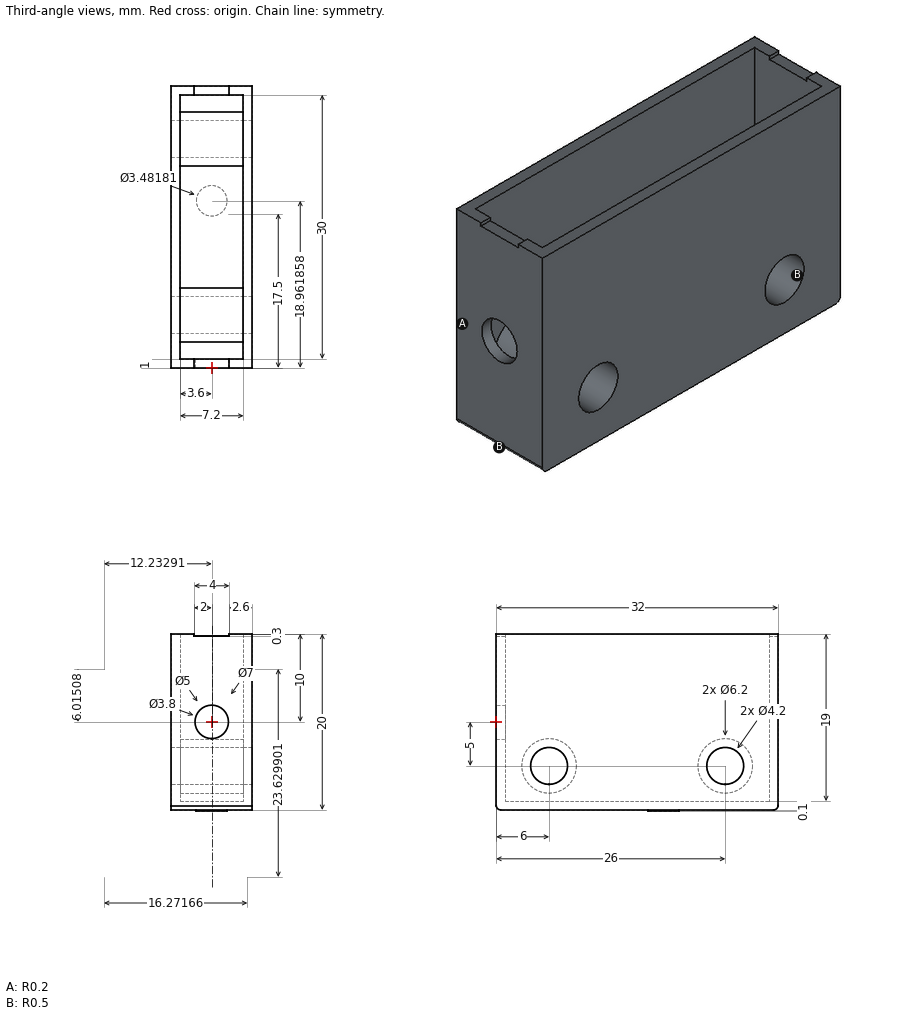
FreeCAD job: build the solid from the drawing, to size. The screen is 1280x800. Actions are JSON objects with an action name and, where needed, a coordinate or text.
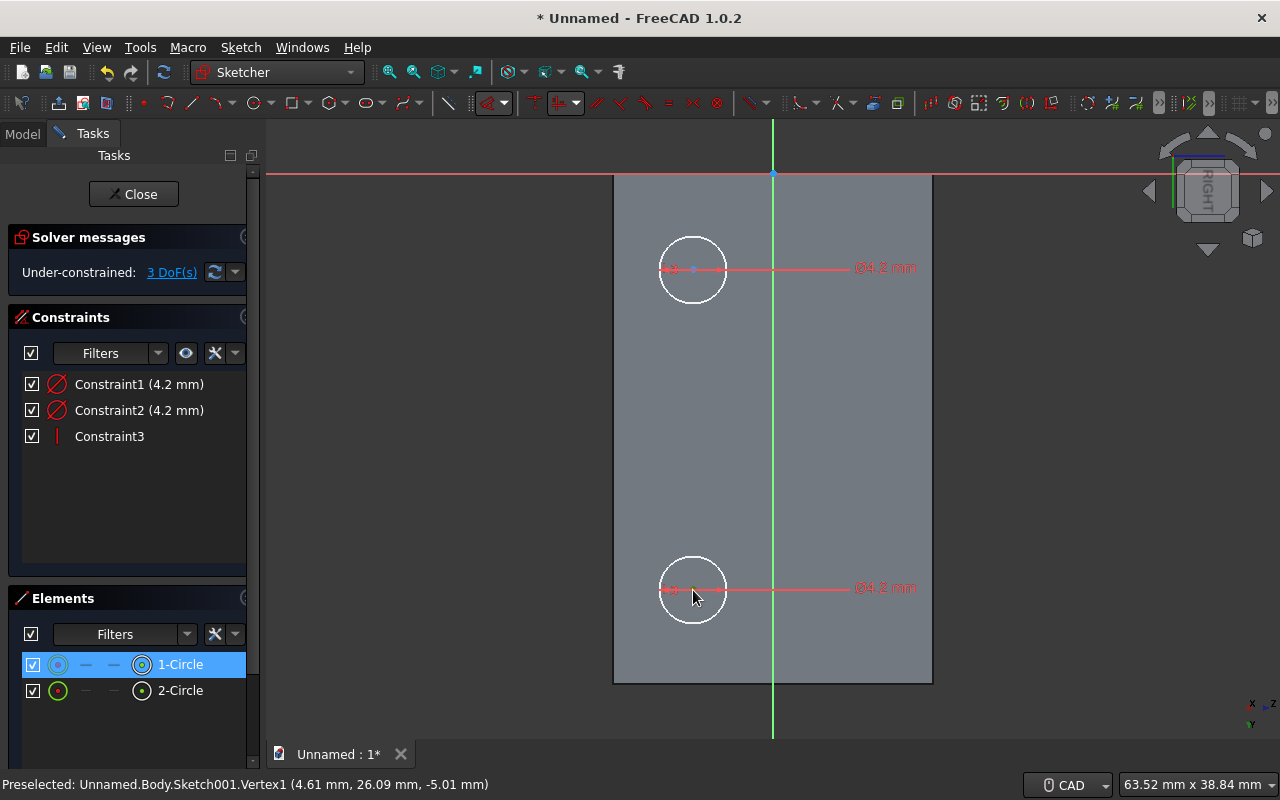
{"action": "key", "text": "l"}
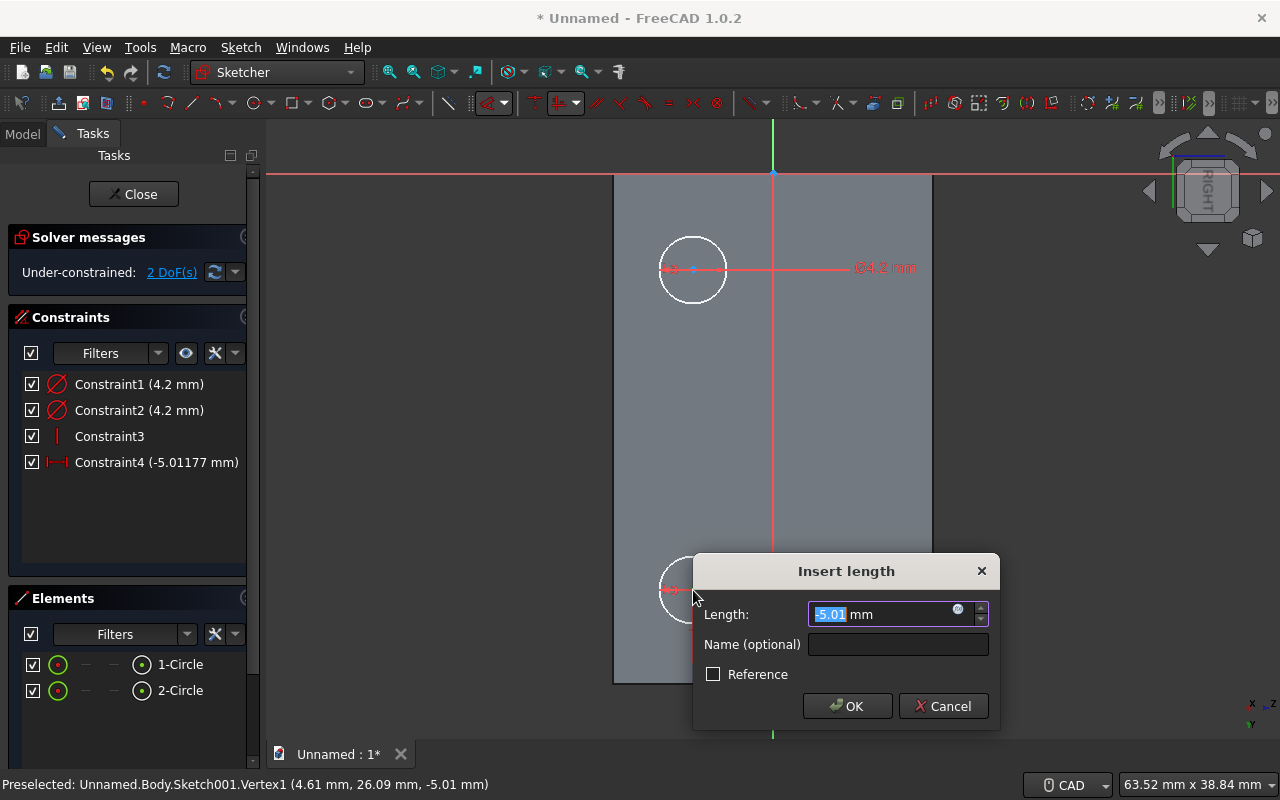
{"action": "type", "text": "-5"}
{"action": "key", "text": "Return"}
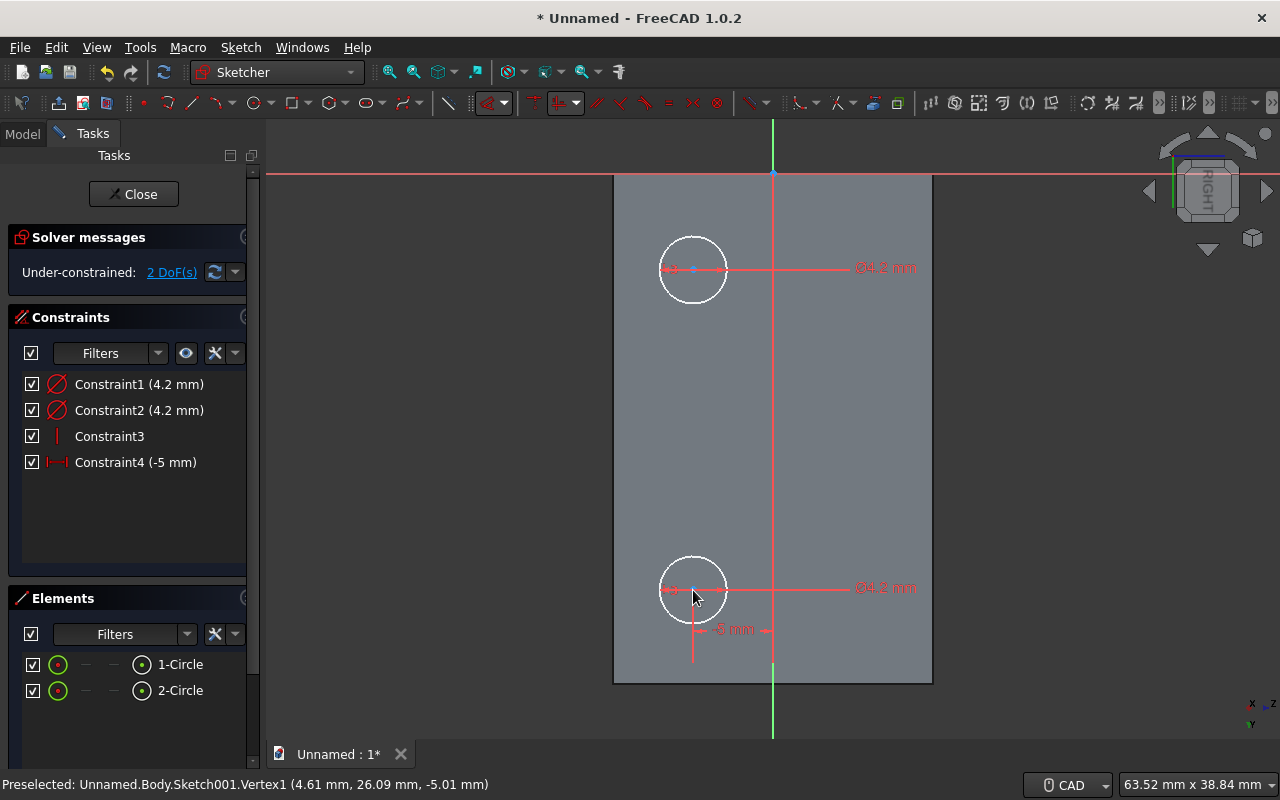
{"action": "left_click", "coordinate": [693, 270]}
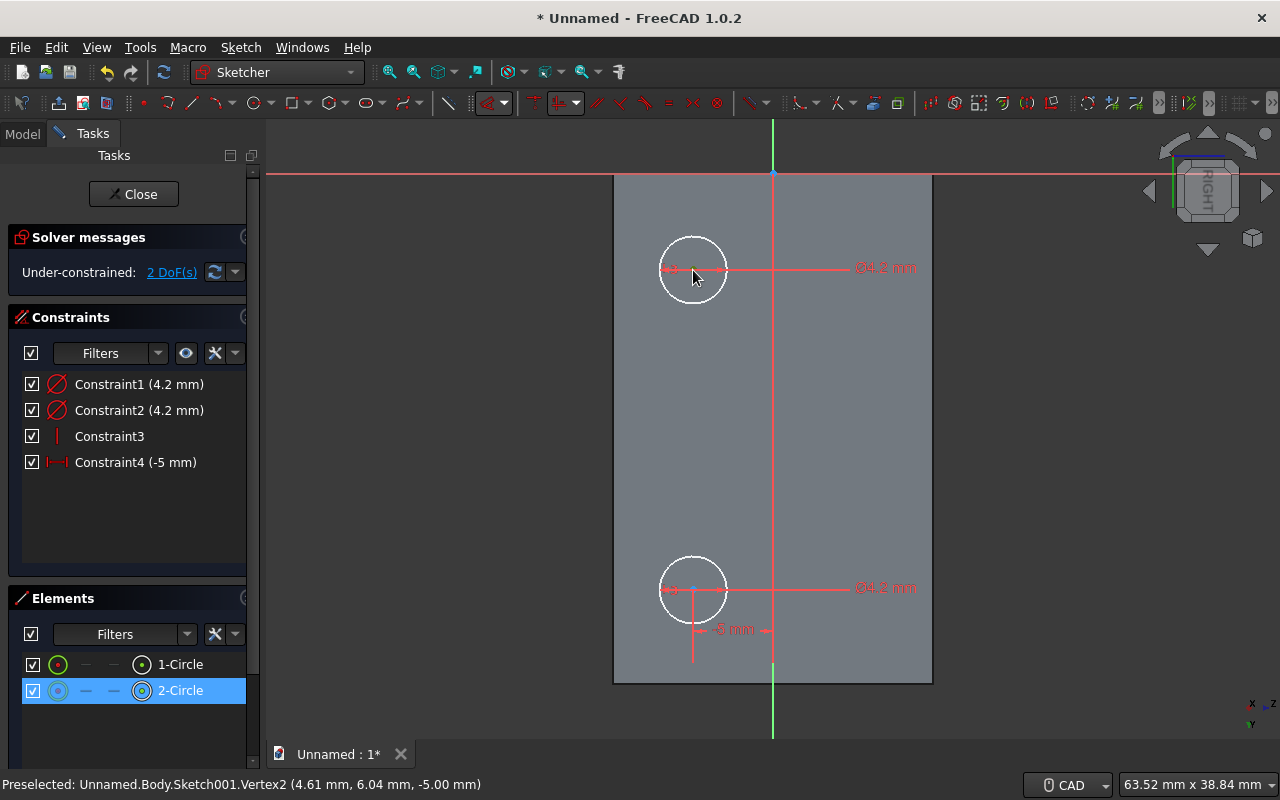
{"action": "left_click", "coordinate": [506, 104]}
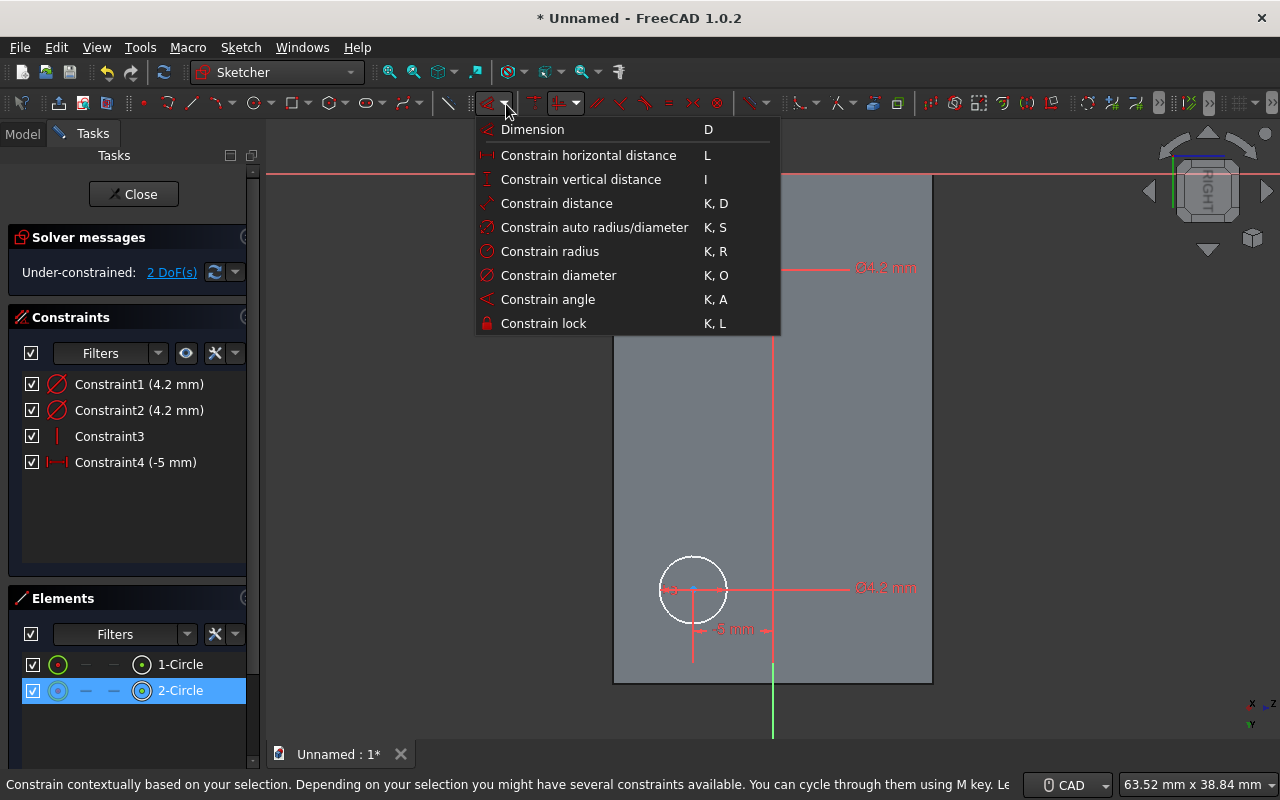
{"action": "left_click", "coordinate": [628, 179]}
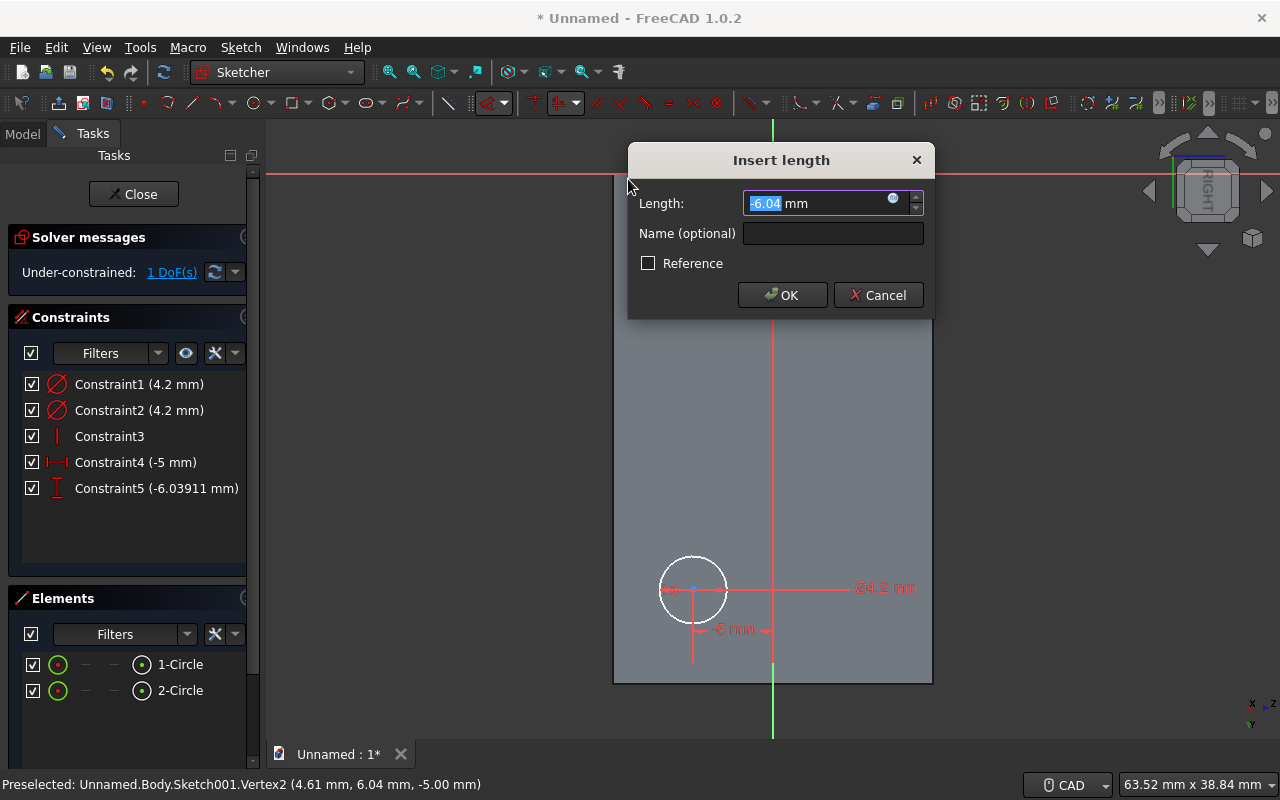
{"action": "type", "text": "-6"}
{"action": "key", "text": "Return"}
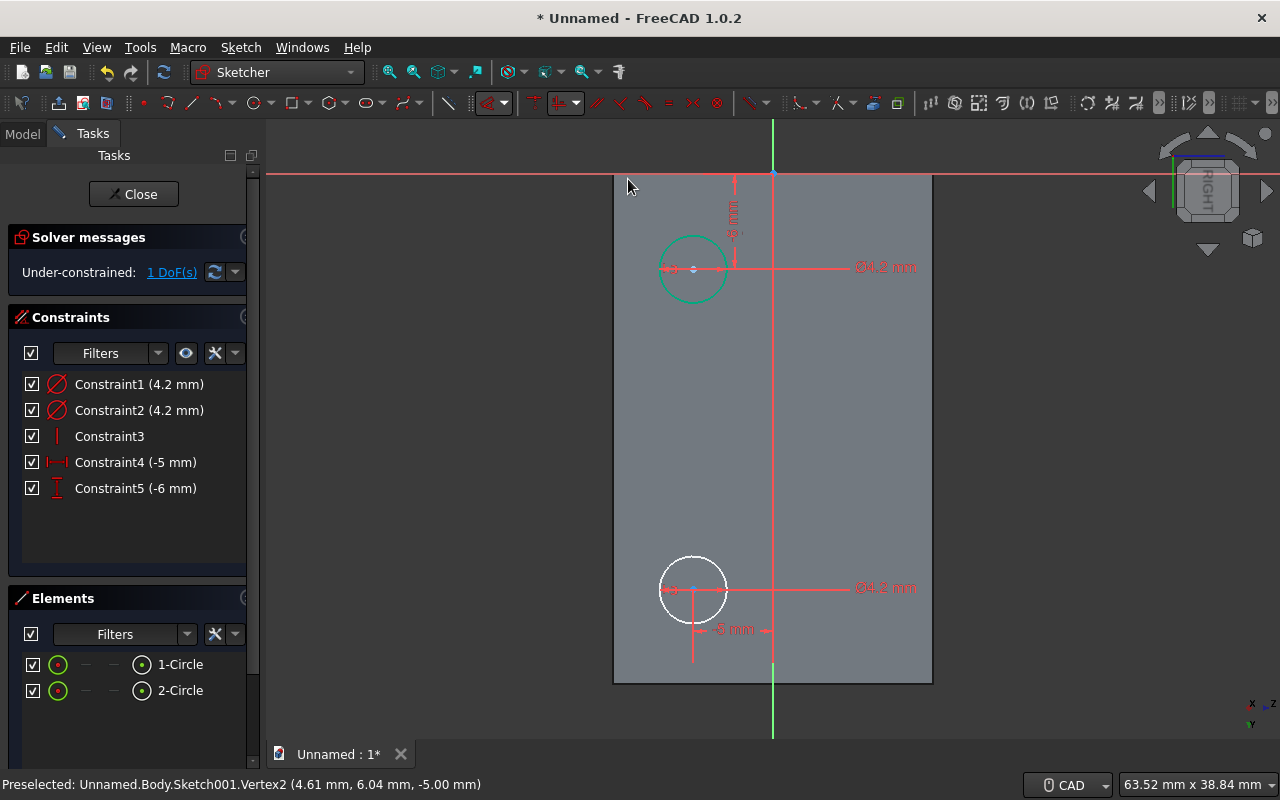
{"action": "left_click", "coordinate": [693, 590]}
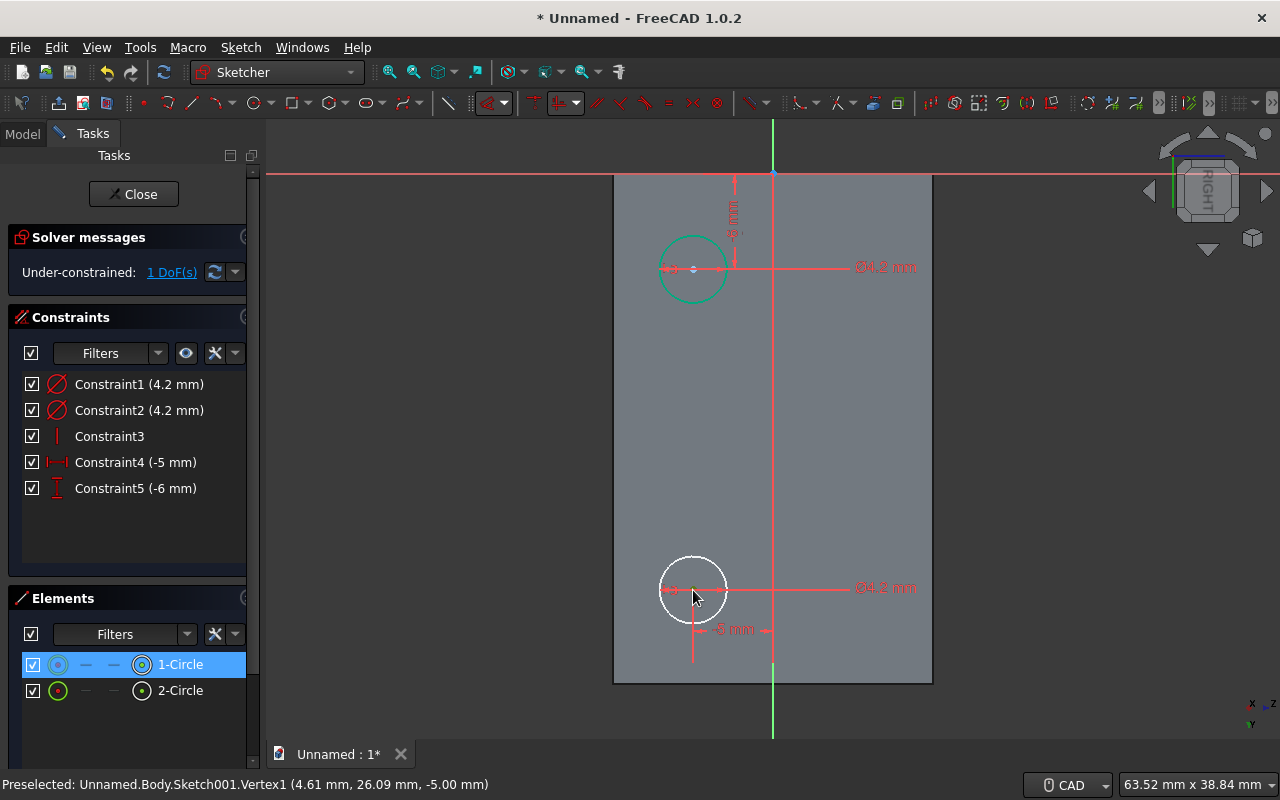
{"action": "left_click", "coordinate": [506, 104]}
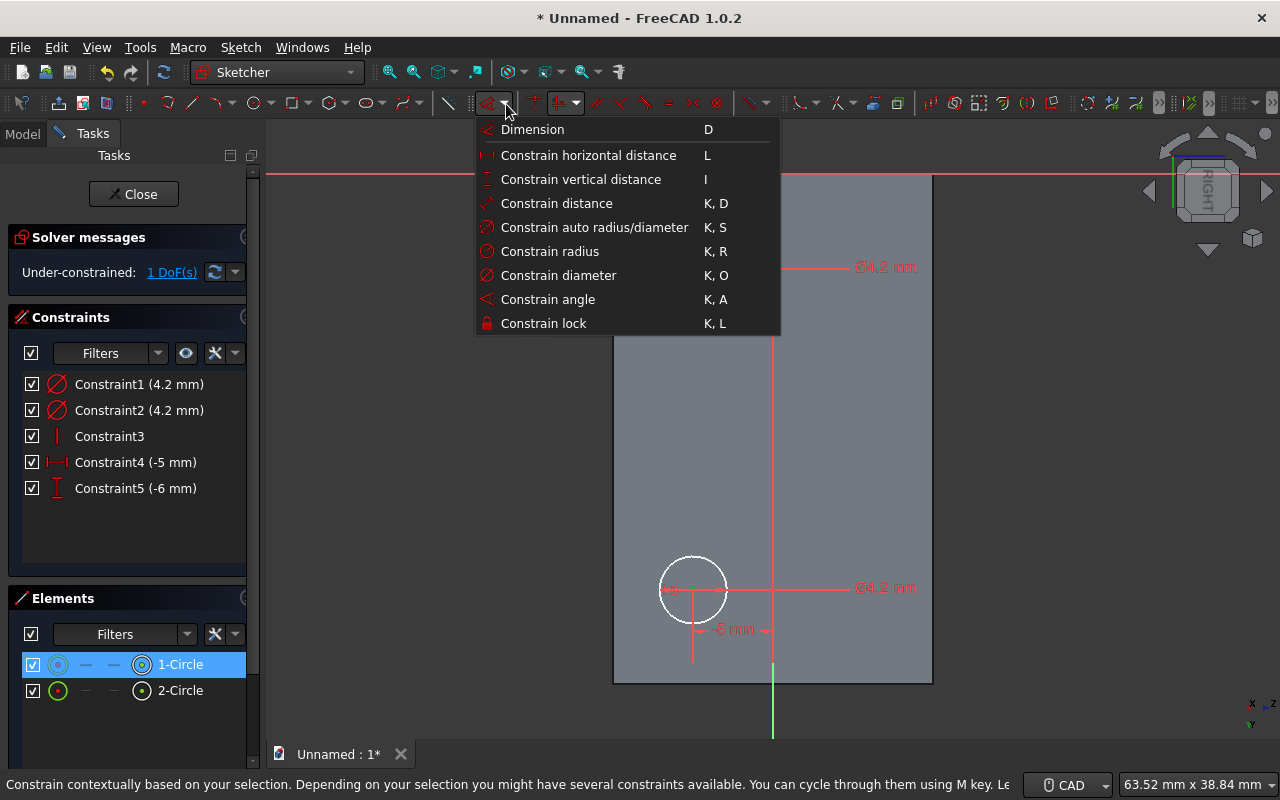
{"action": "left_click", "coordinate": [628, 179]}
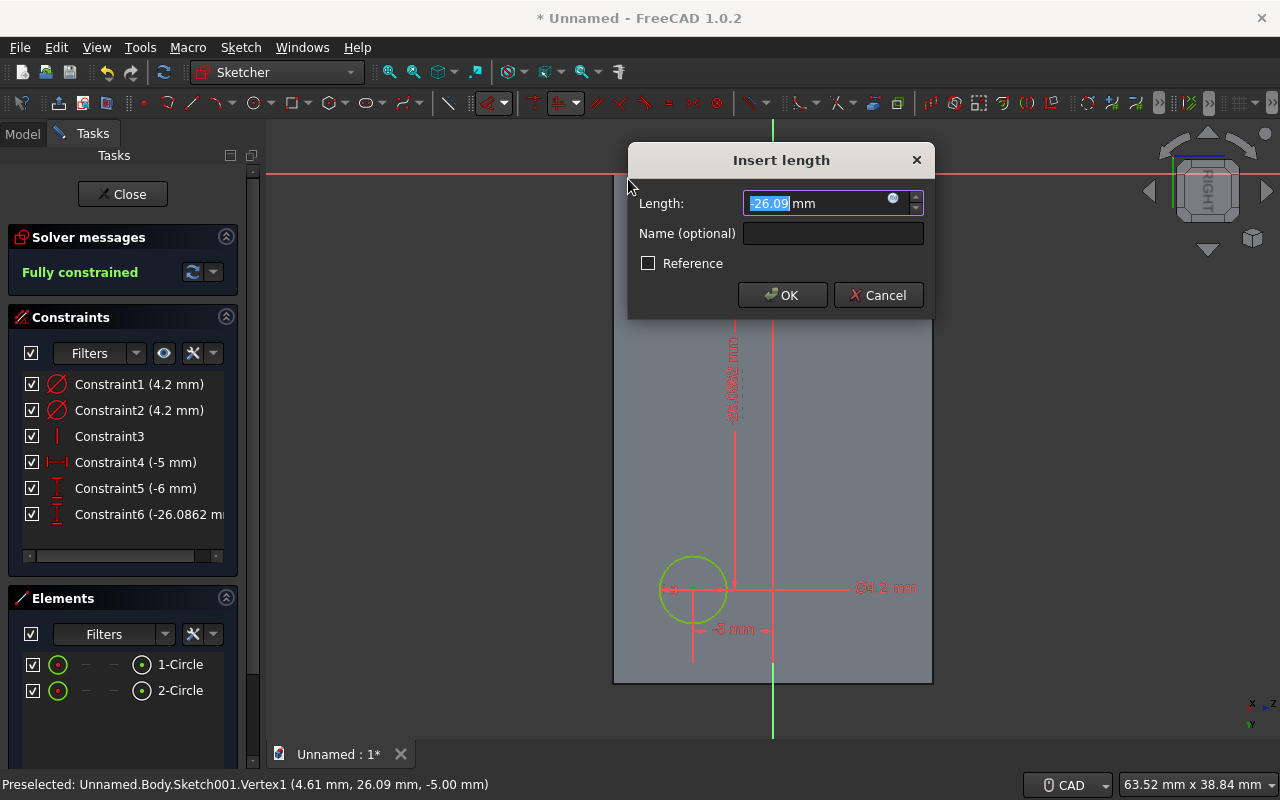
{"action": "type", "text": "-26"}
{"action": "key", "text": "Return"}